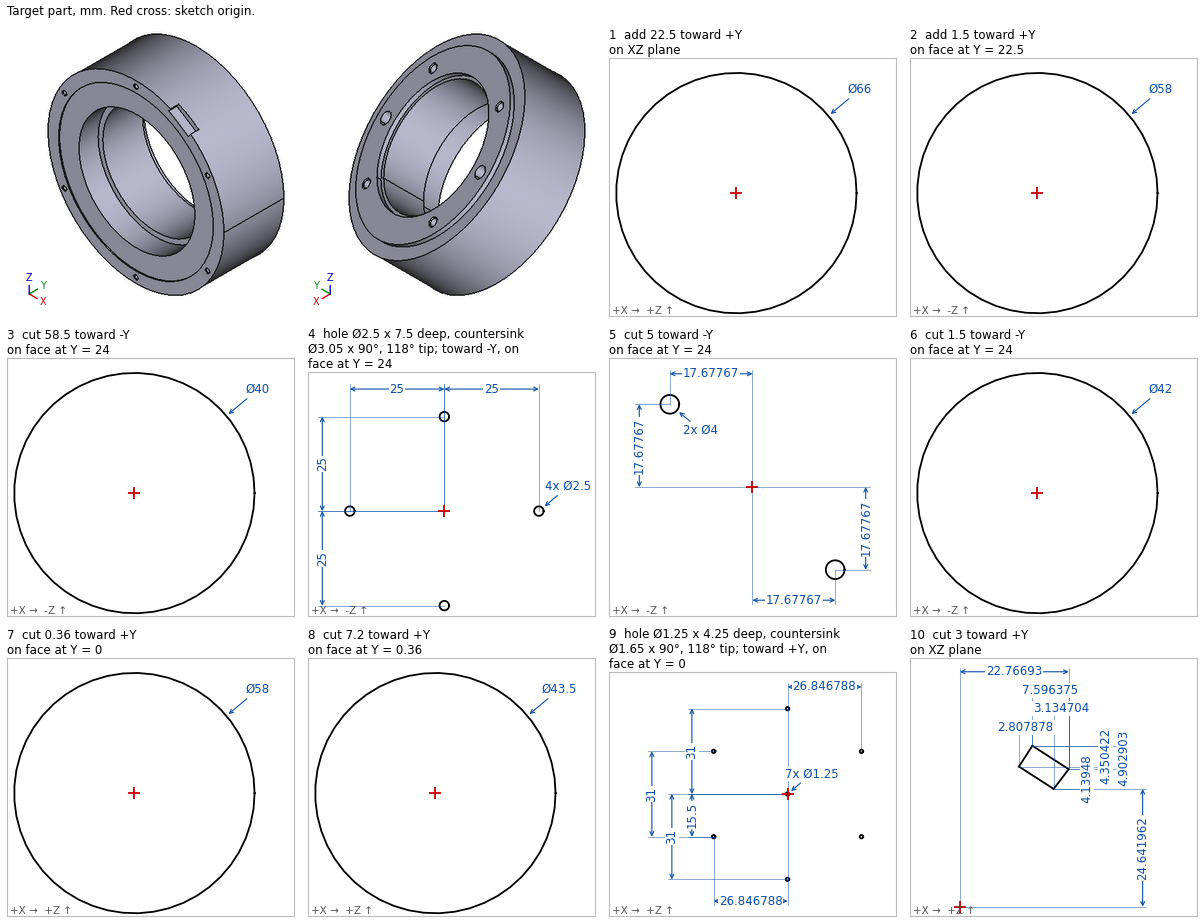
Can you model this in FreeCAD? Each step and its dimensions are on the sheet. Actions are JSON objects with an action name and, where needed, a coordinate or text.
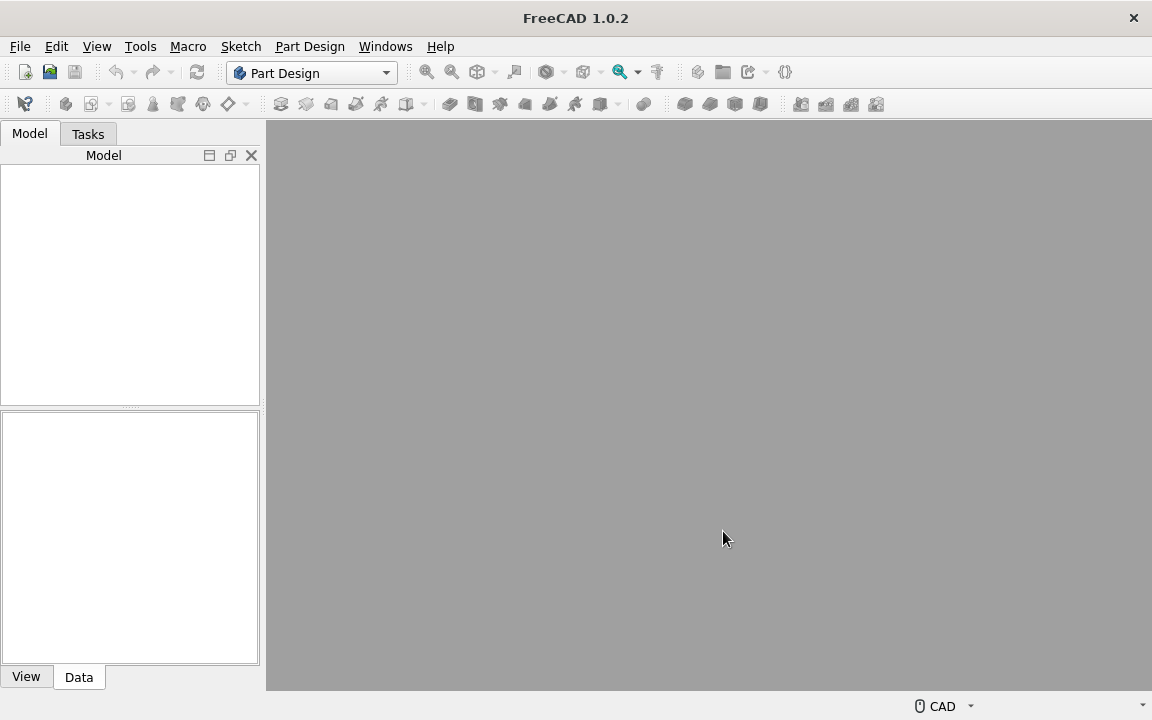
{"action": "left_click", "coordinate": [25, 72]}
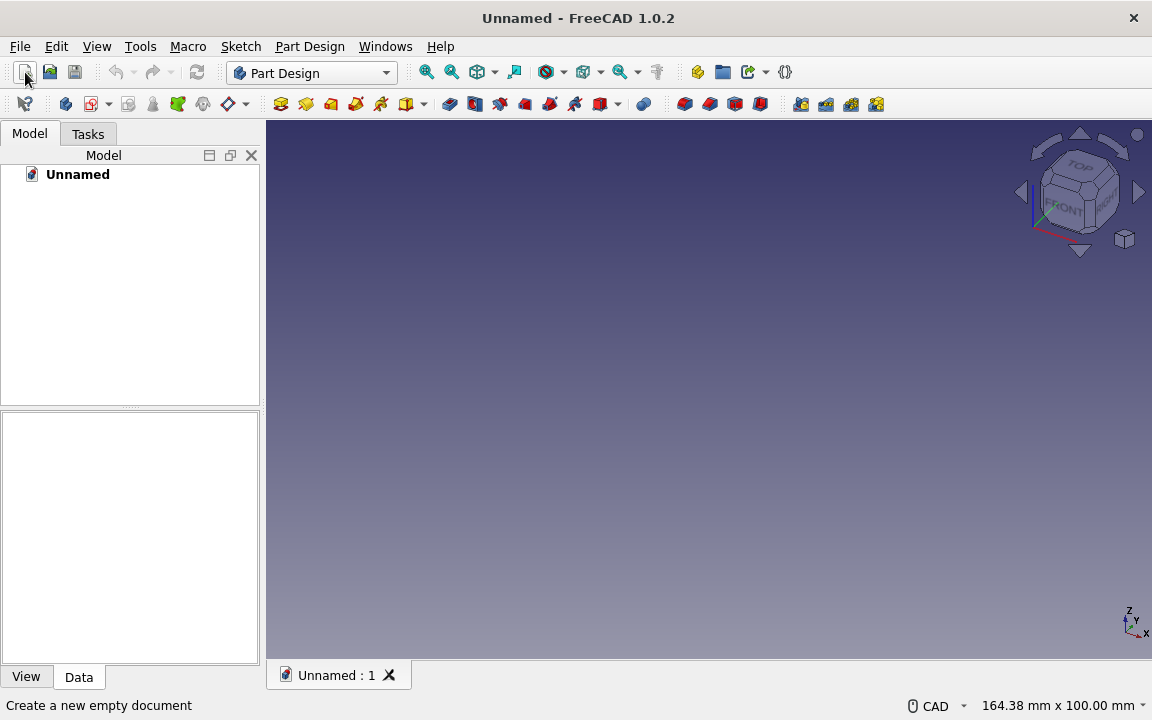
{"action": "left_click", "coordinate": [90, 104]}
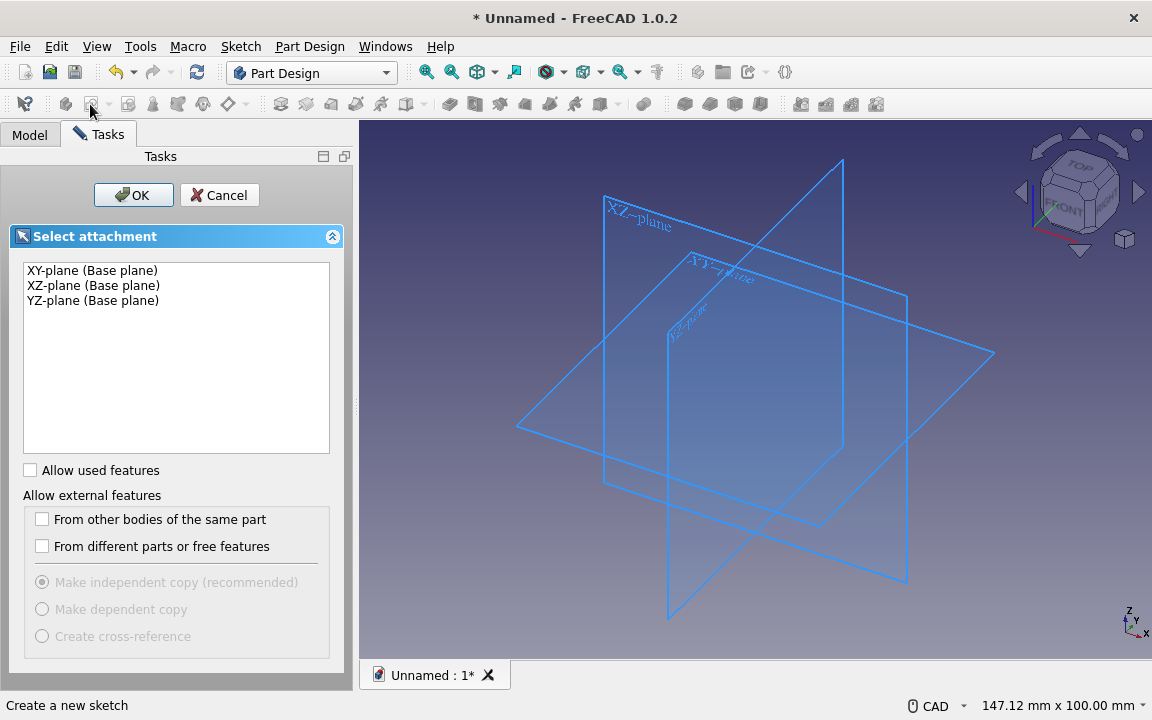
{"action": "left_click", "coordinate": [84, 286]}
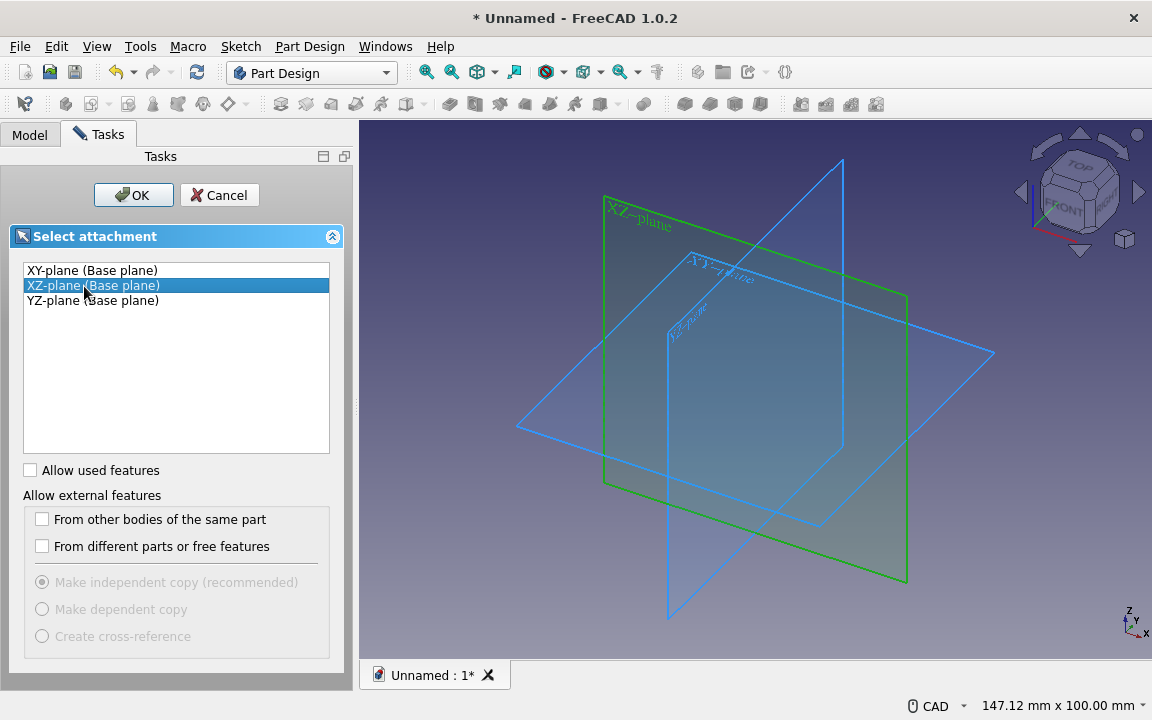
{"action": "left_click", "coordinate": [134, 195]}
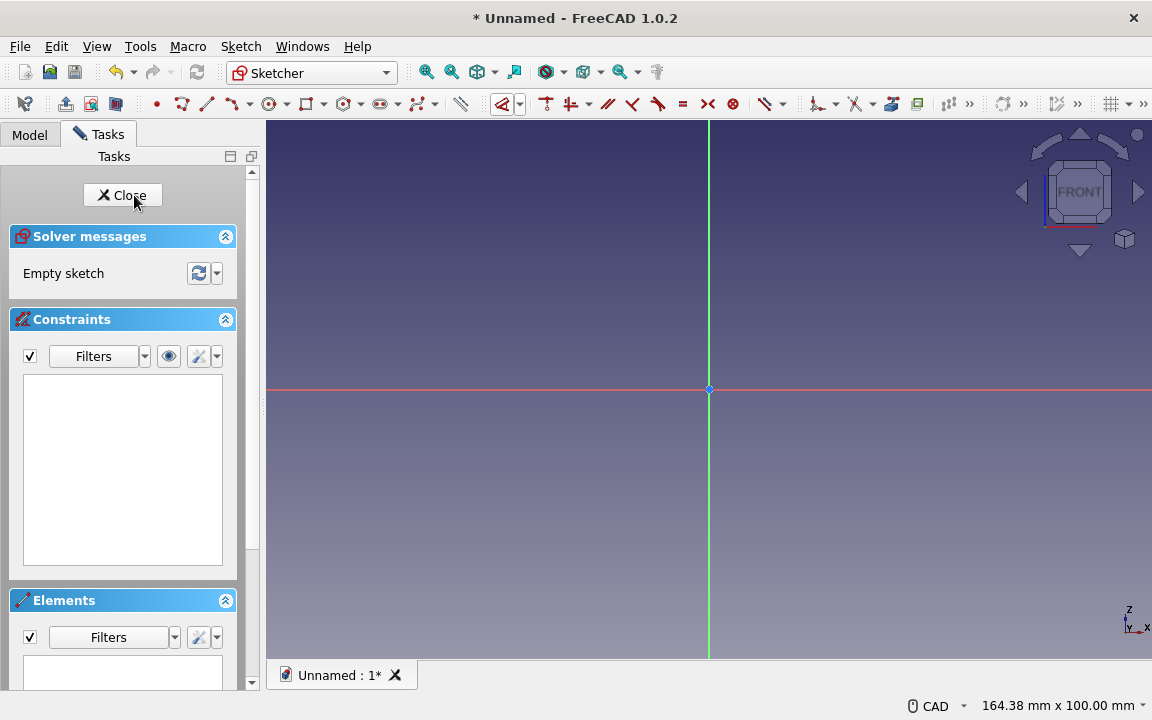
{"action": "left_click", "coordinate": [268, 104]}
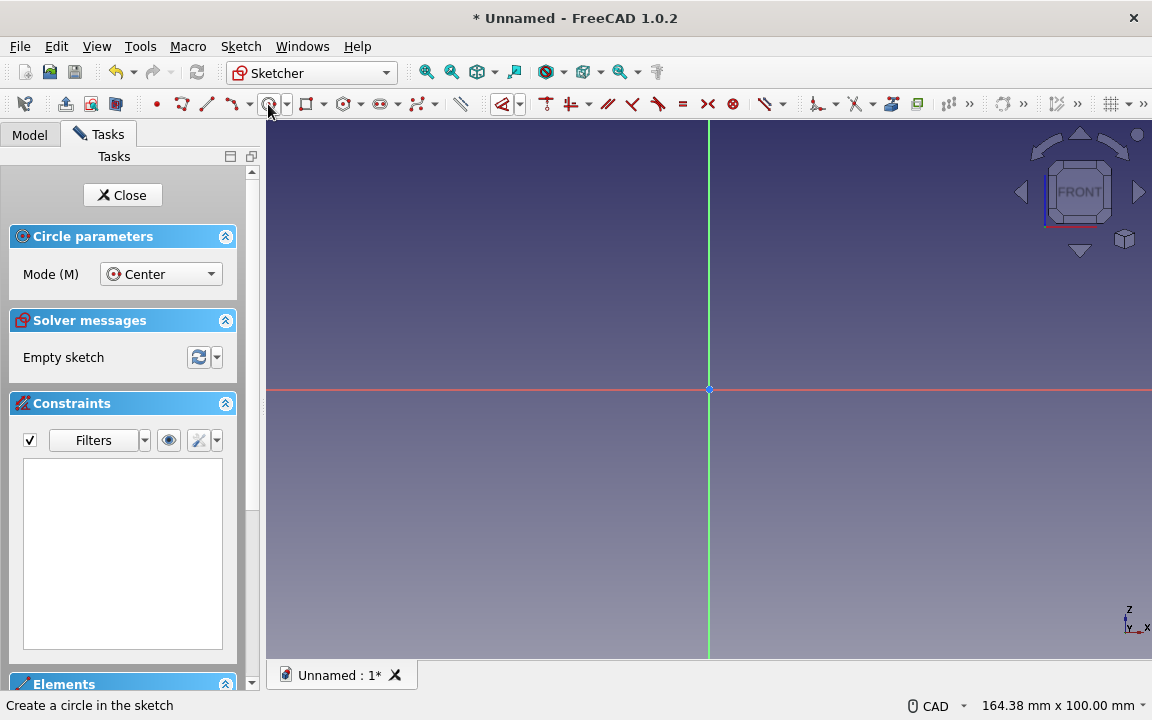
{"action": "left_click", "coordinate": [709, 390]}
{"action": "left_click", "coordinate": [835, 264]}
{"action": "key", "text": "Escape"}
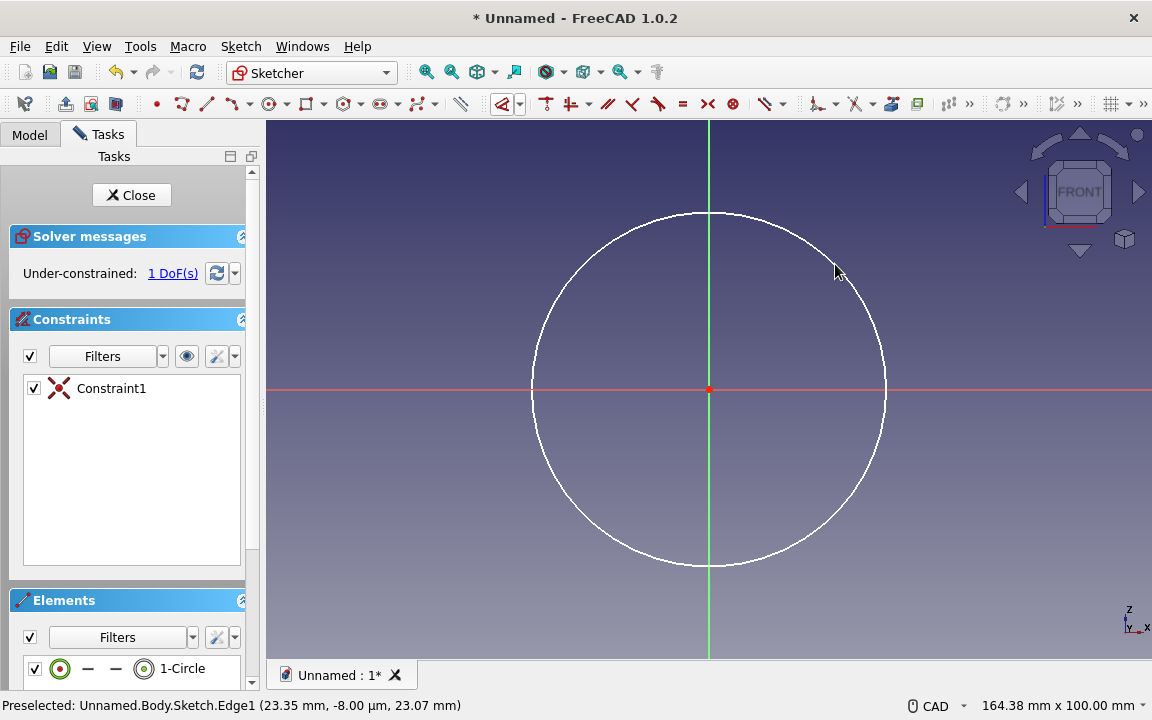
{"action": "left_click", "coordinate": [834, 264]}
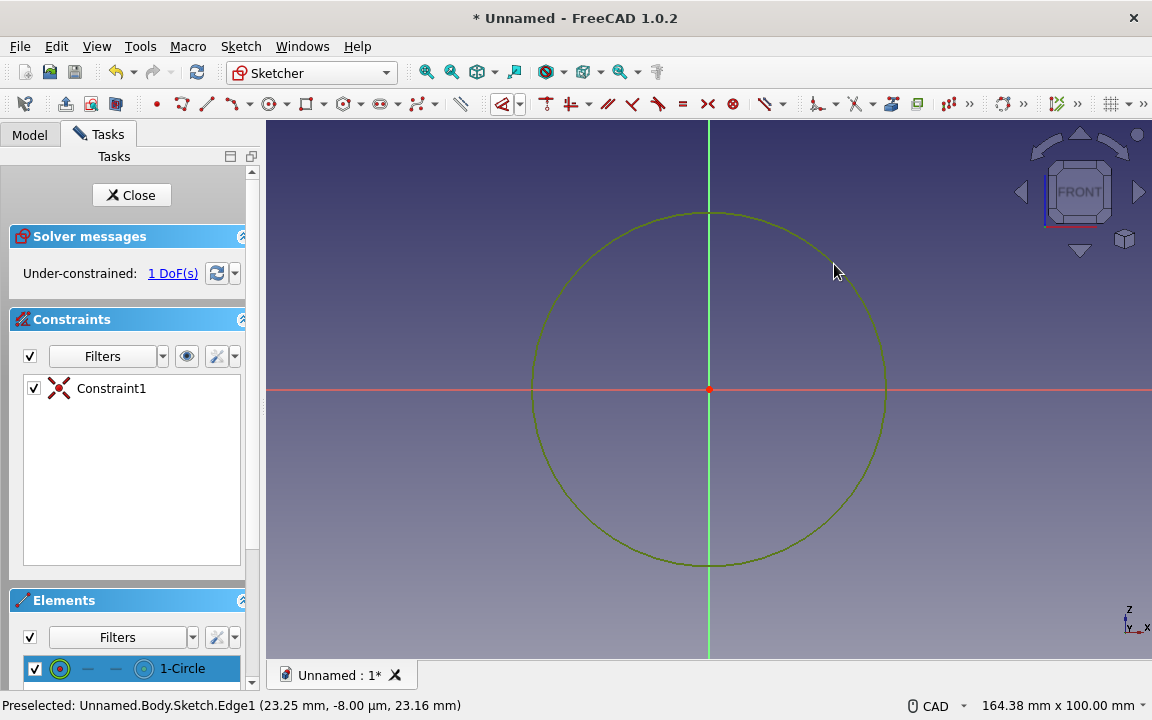
{"action": "left_click", "coordinate": [520, 104]}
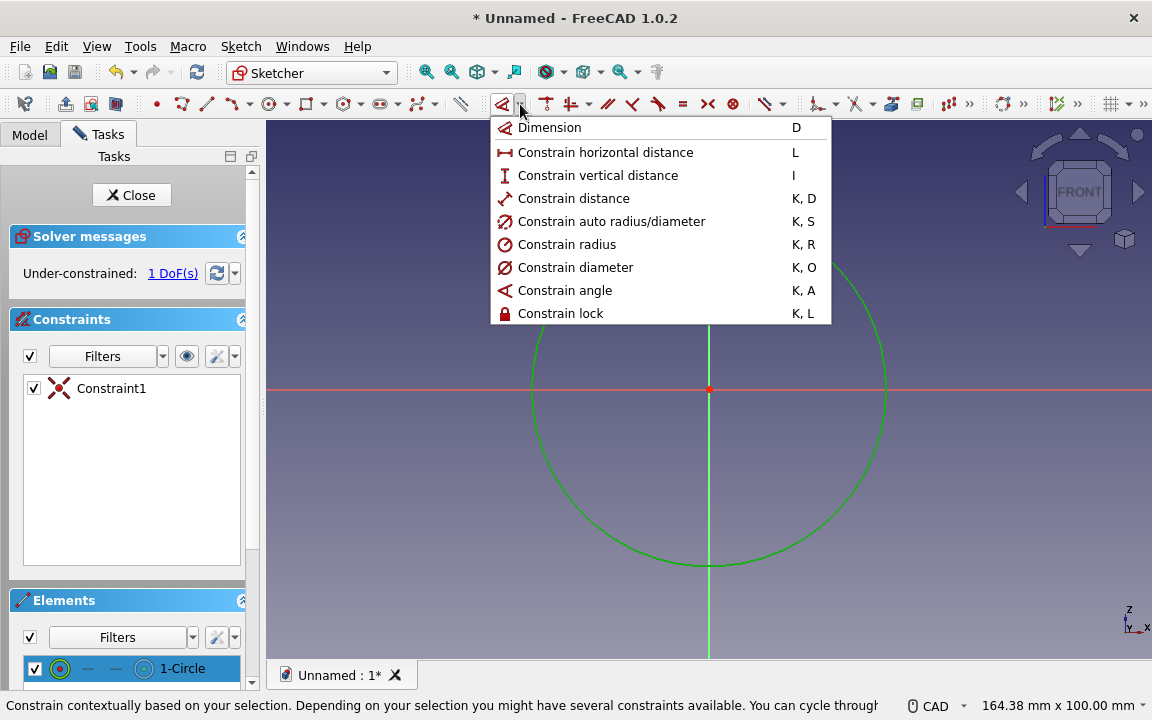
{"action": "left_click", "coordinate": [661, 268]}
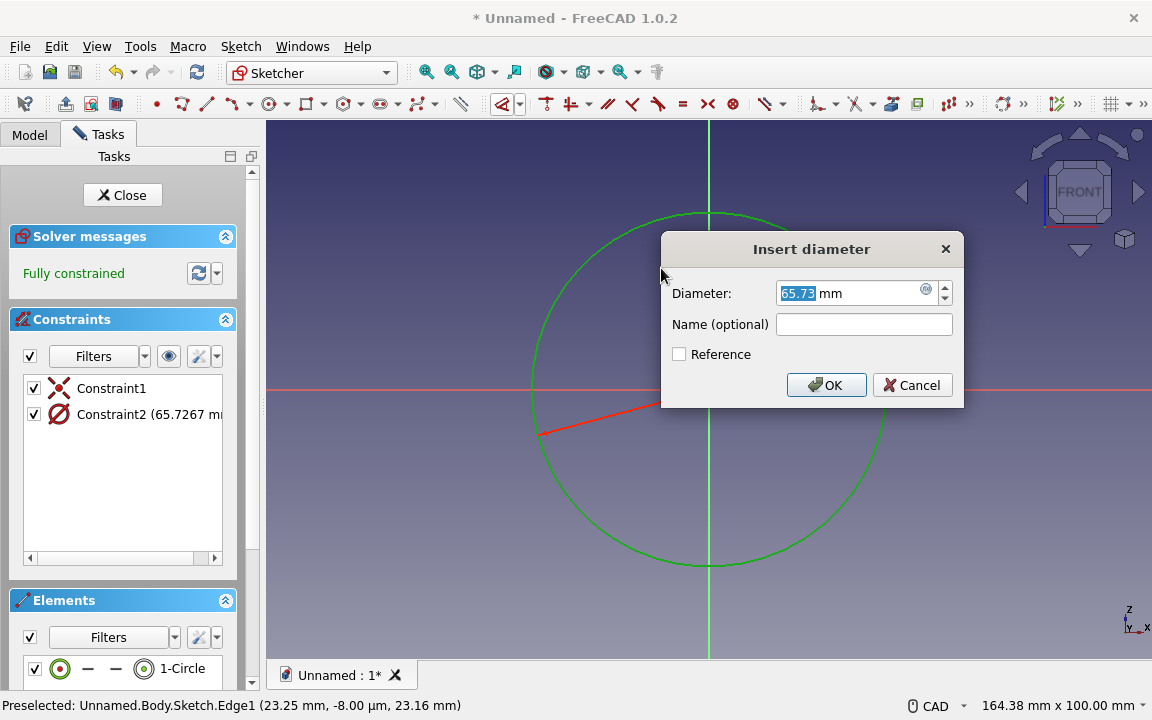
{"action": "type", "text": "66"}
{"action": "key", "text": "Return"}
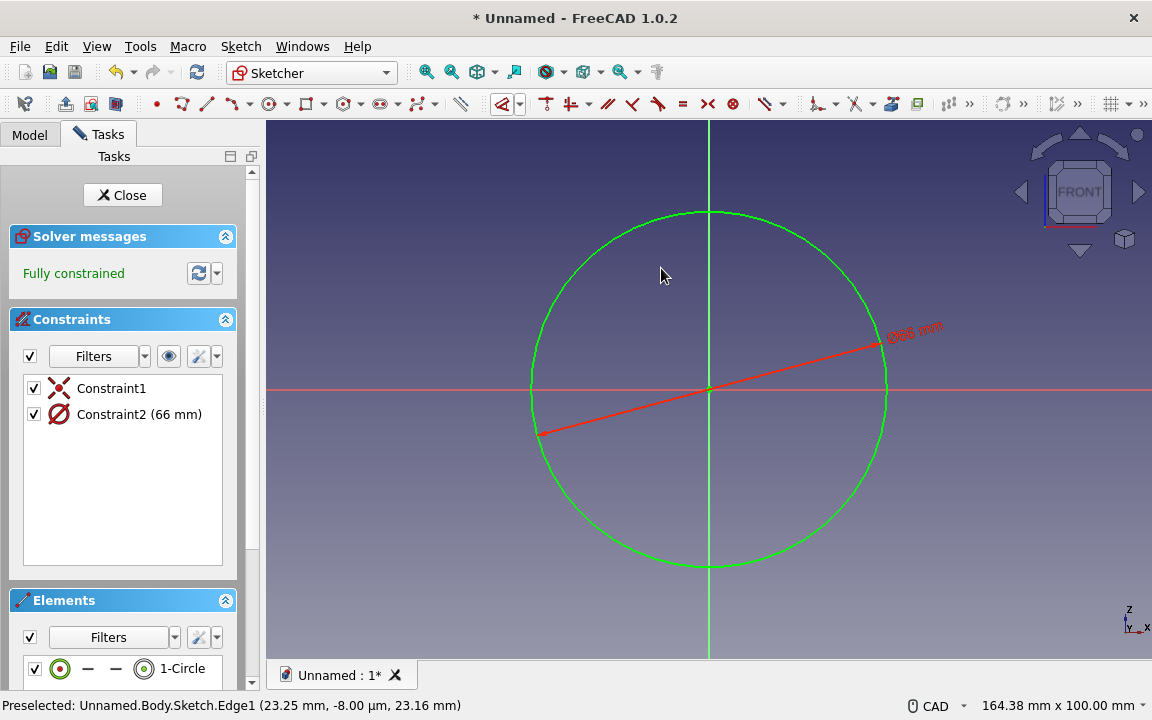
{"action": "left_click", "coordinate": [123, 195]}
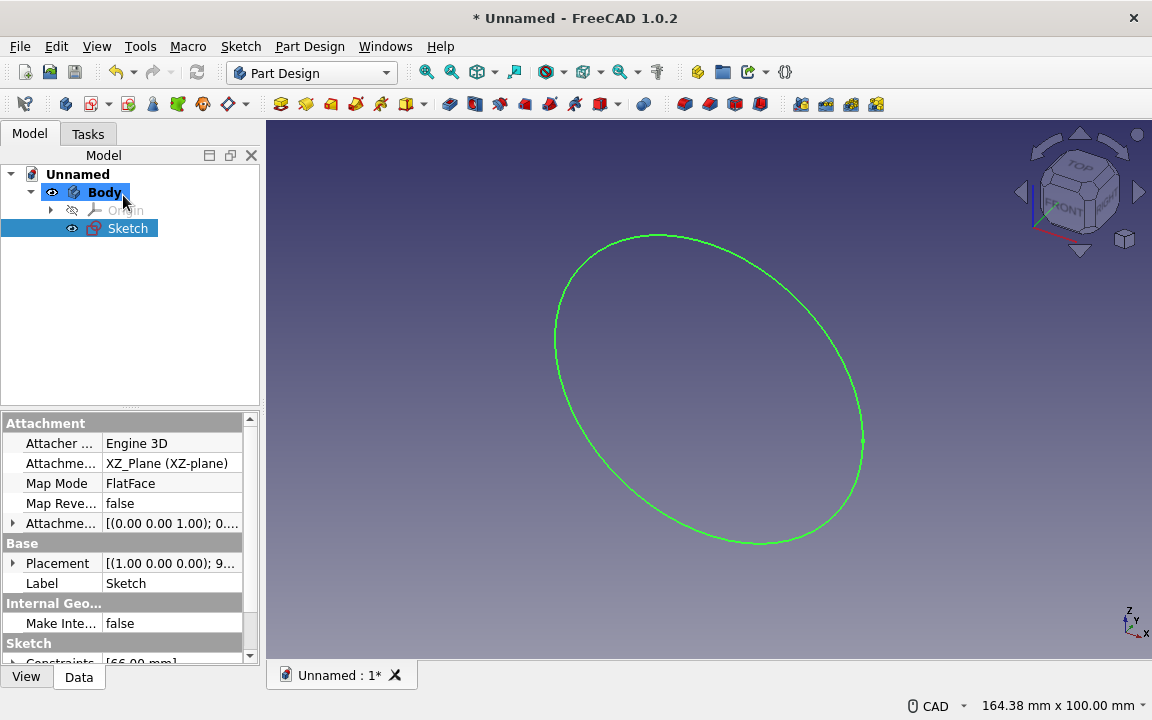
{"action": "left_click", "coordinate": [281, 104]}